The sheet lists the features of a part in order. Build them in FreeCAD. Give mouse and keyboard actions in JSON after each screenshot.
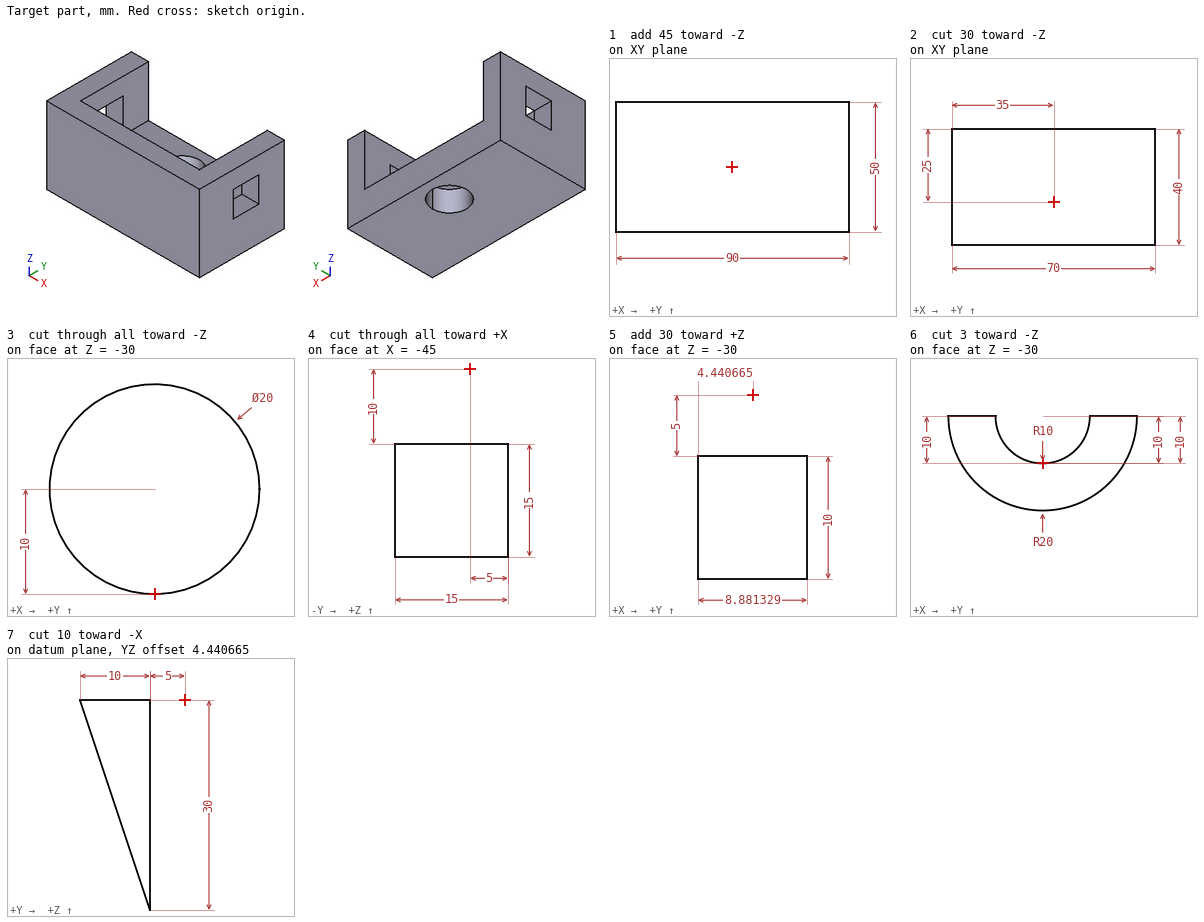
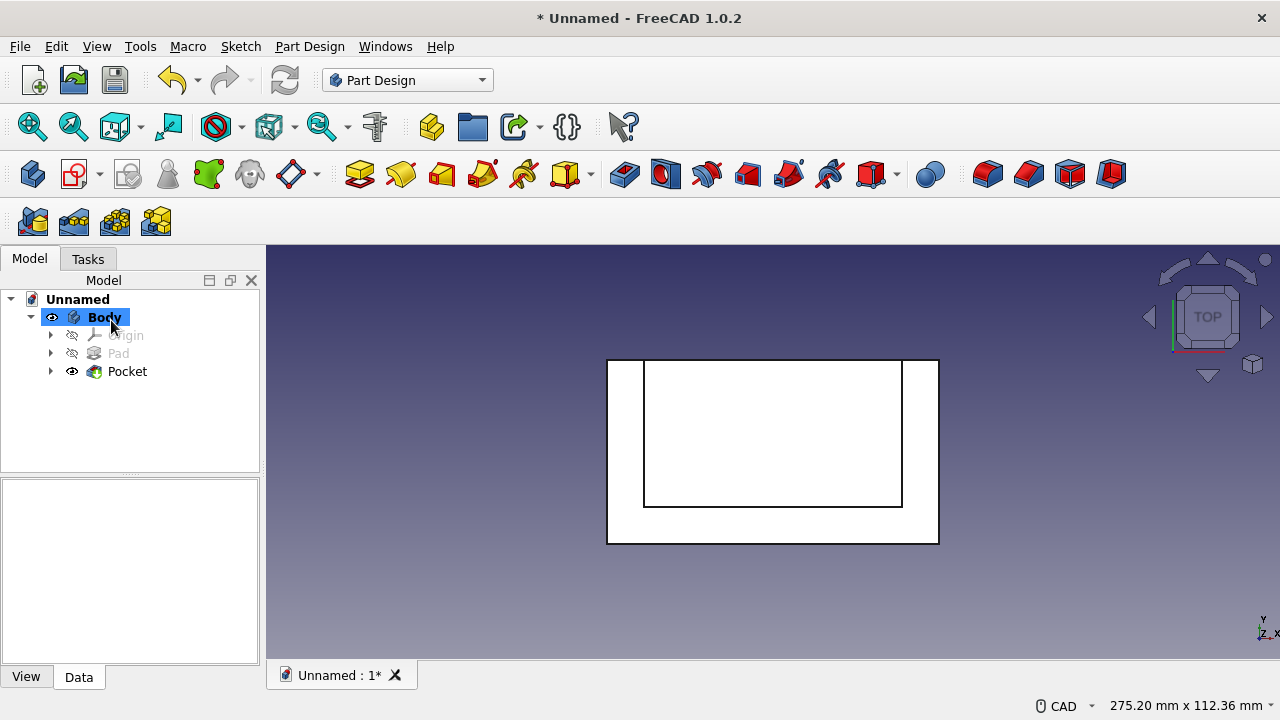
{"action": "key", "text": "v f"}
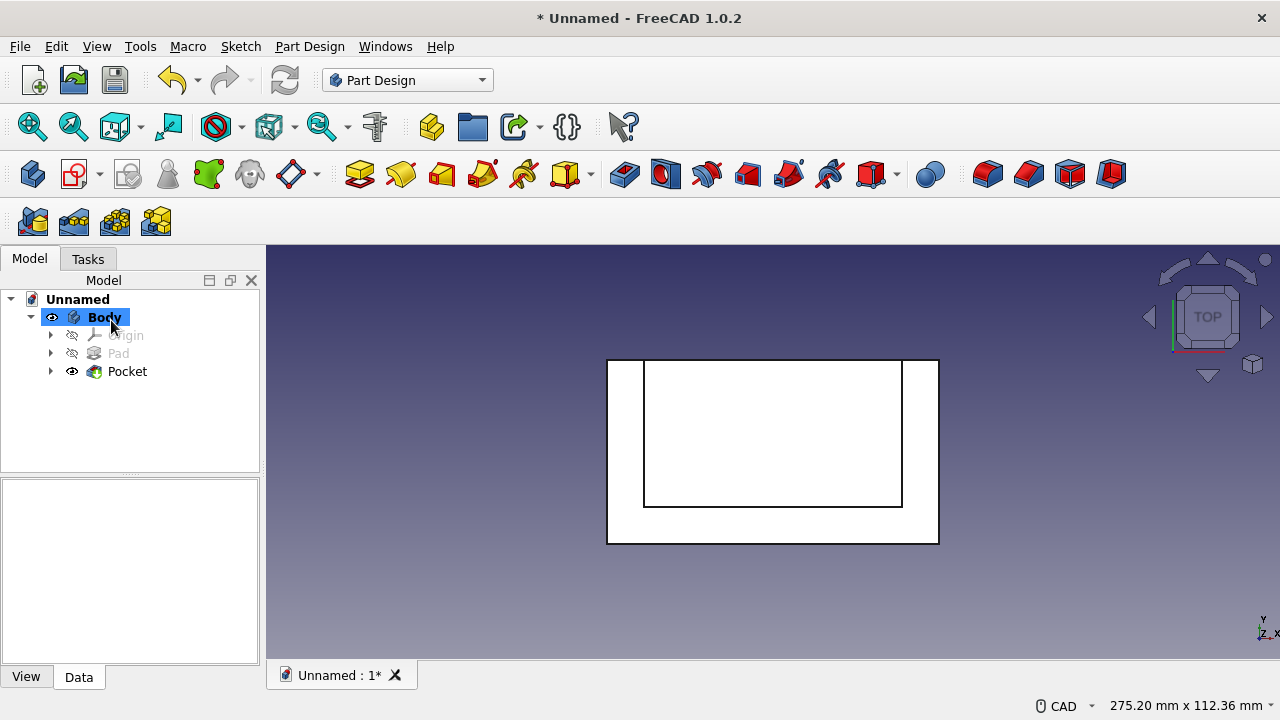
{"action": "left_click", "coordinate": [810, 433]}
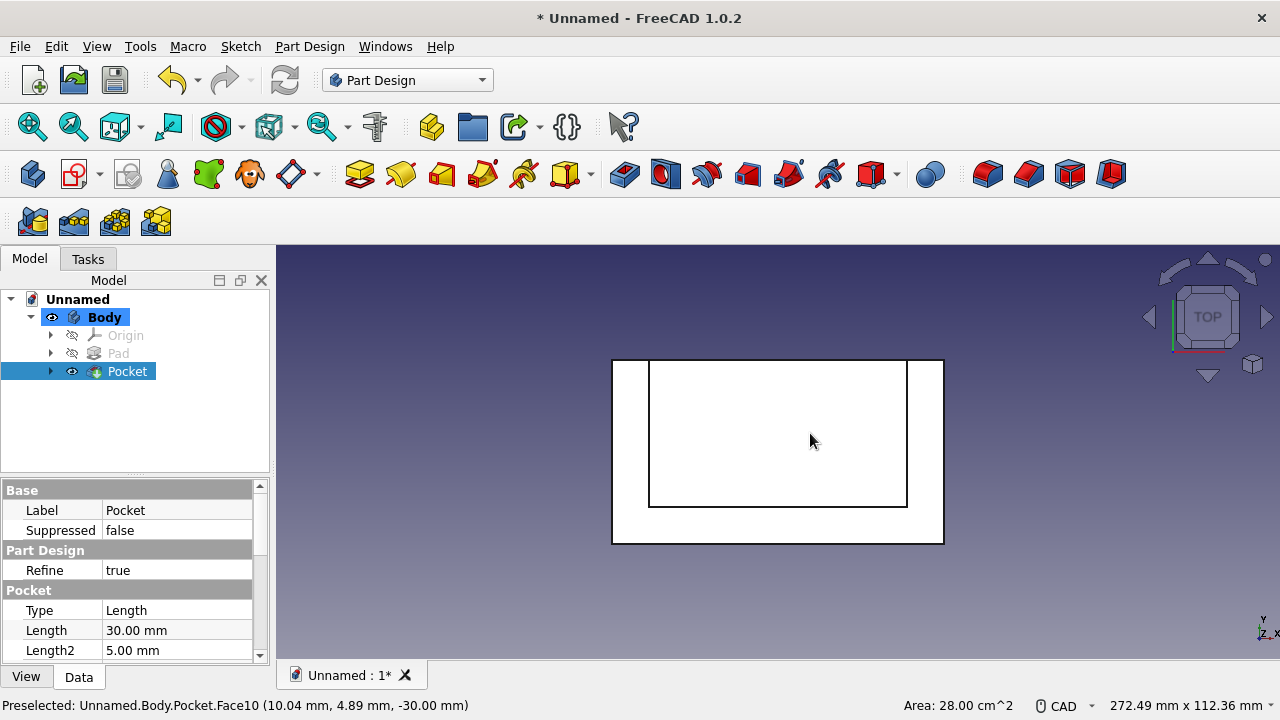
{"action": "left_click", "coordinate": [74, 174]}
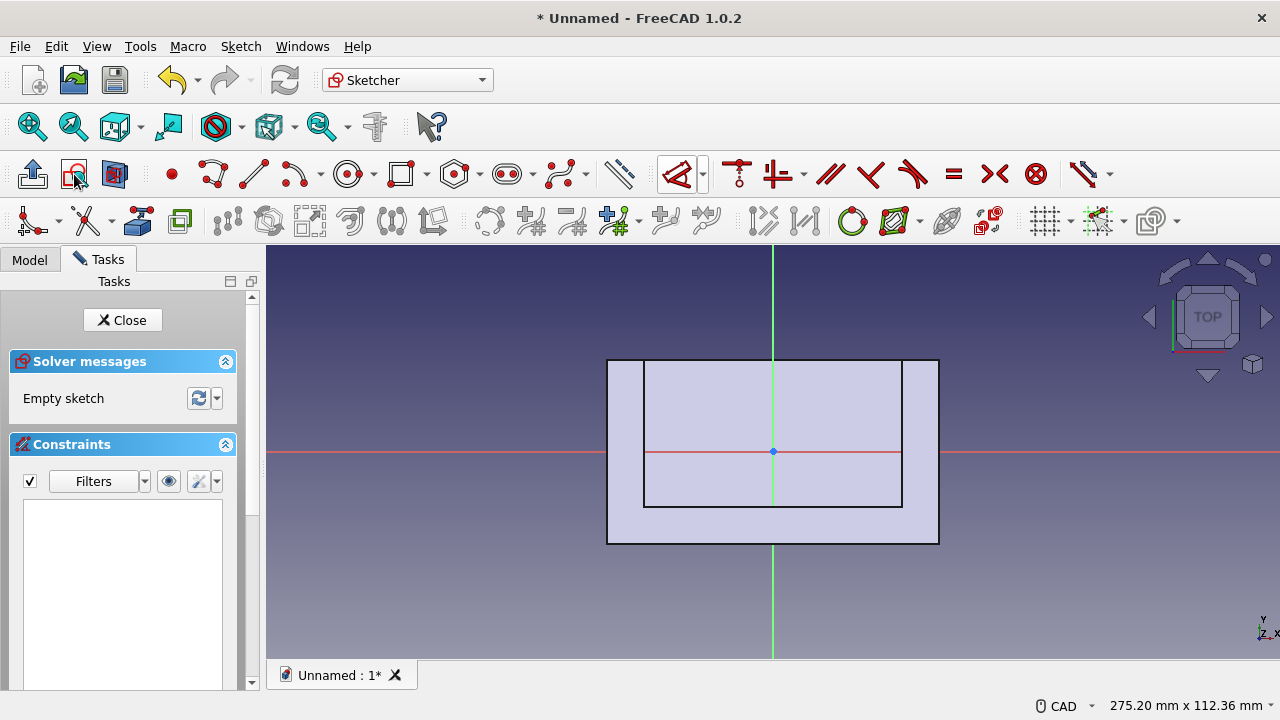
{"action": "scroll", "coordinate": [803, 399], "scroll_direction": "up", "scroll_amount": 6}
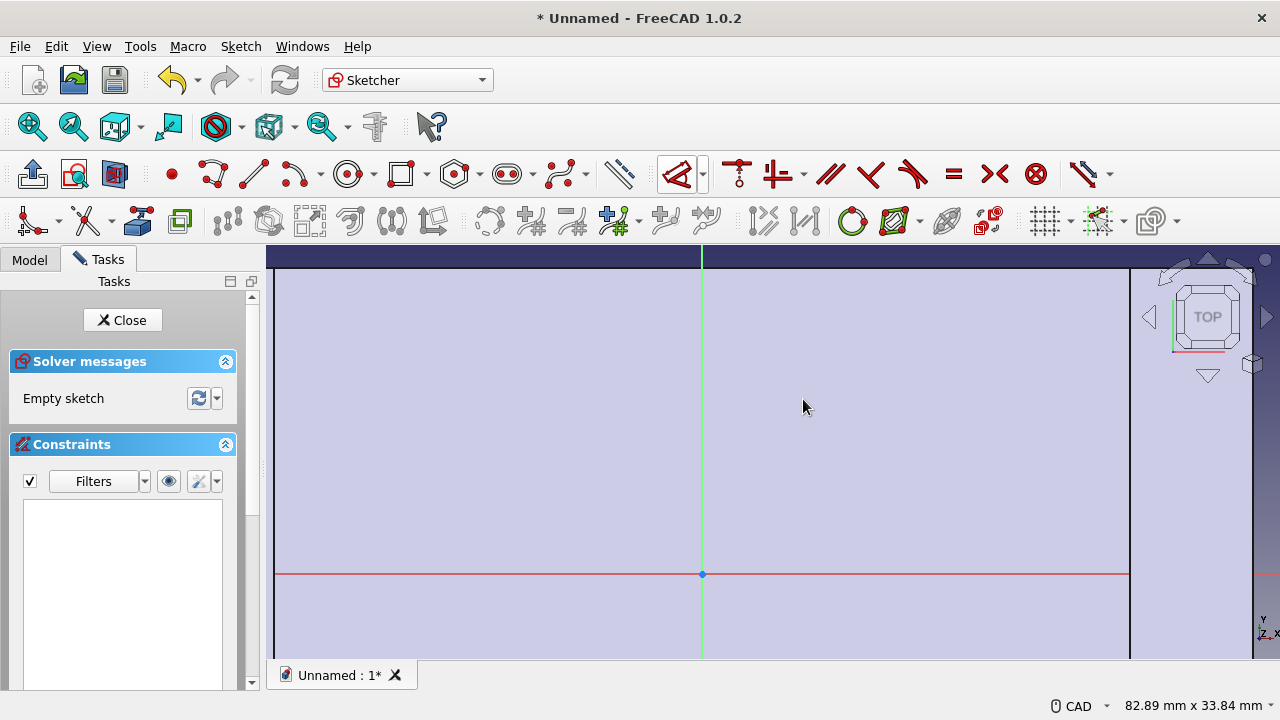
{"action": "key", "text": "g c"}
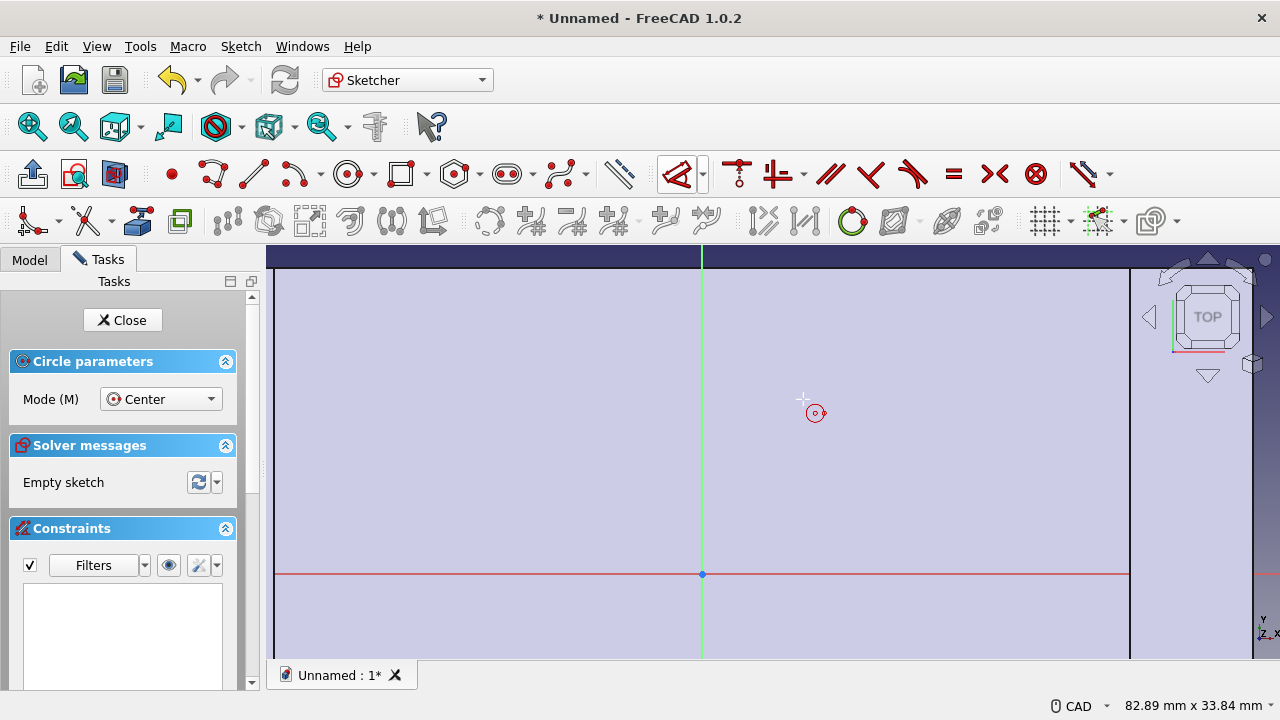
{"action": "left_click", "coordinate": [702, 452]}
{"action": "mouse_move", "coordinate": [789, 365]}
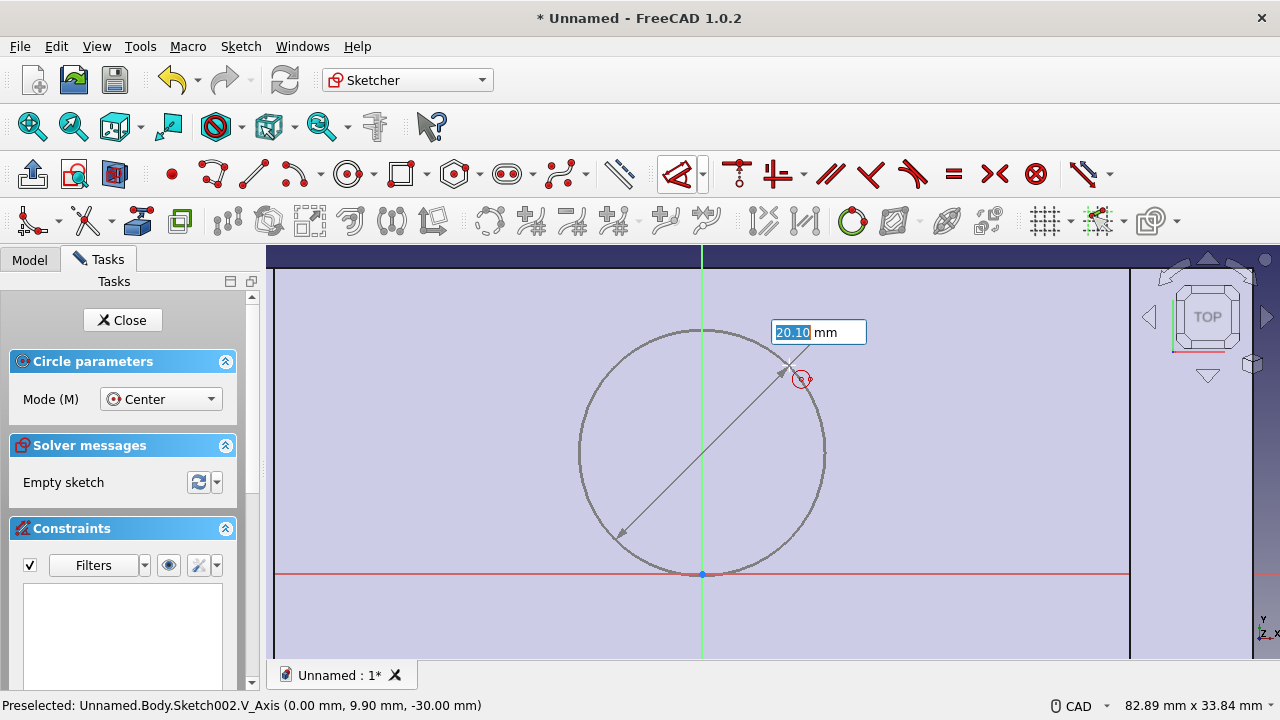
{"action": "type", "text": "20"}
{"action": "key", "text": "Return"}
{"action": "key", "text": "Escape"}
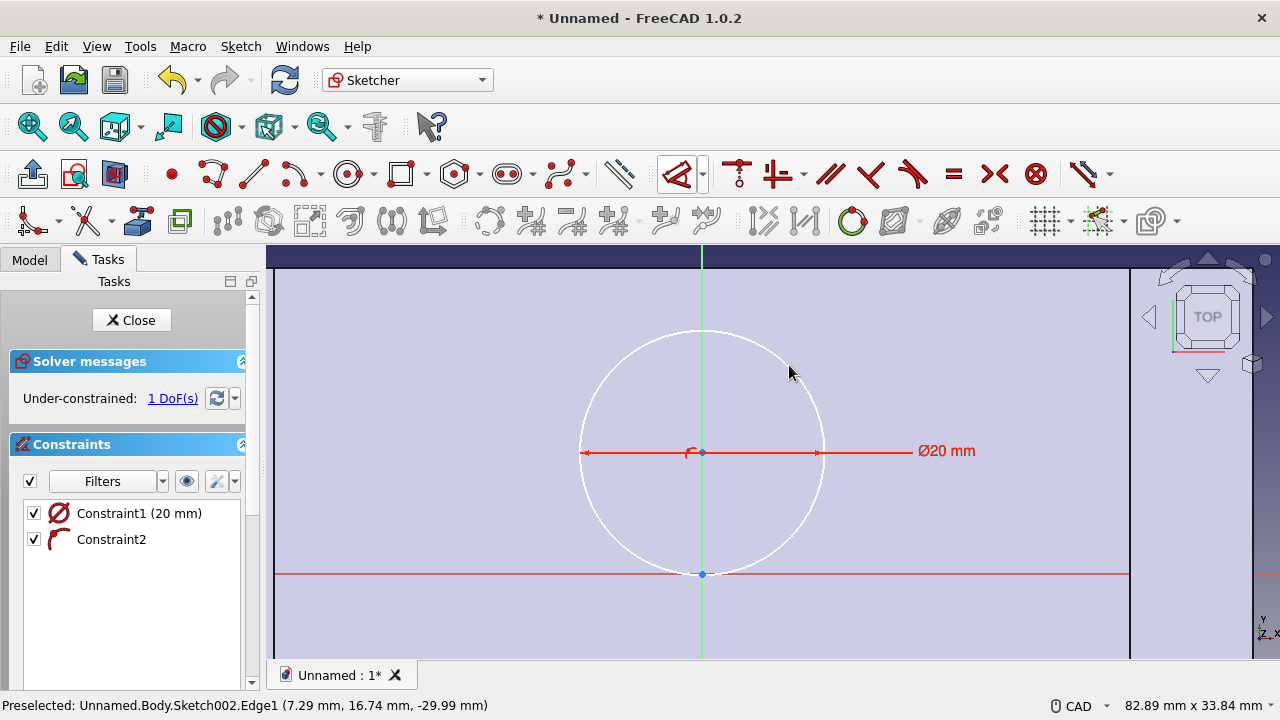
{"action": "left_click", "coordinate": [702, 453]}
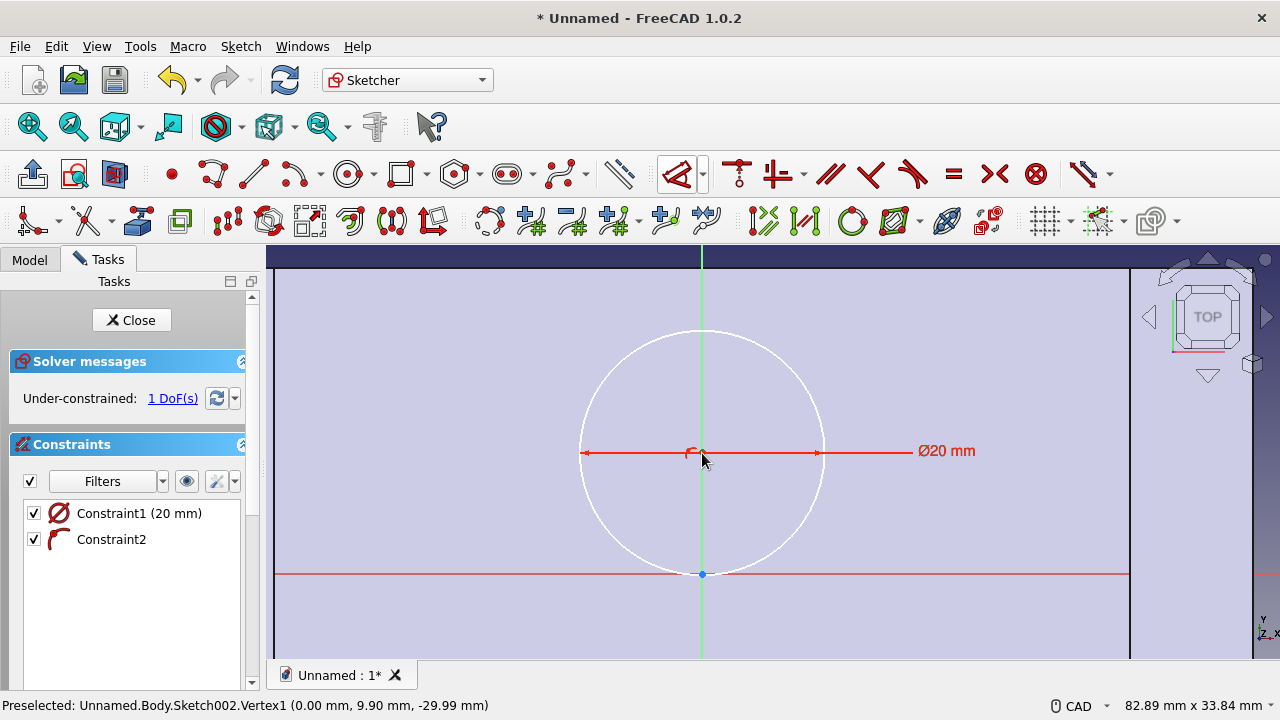
{"action": "key", "text": "i"}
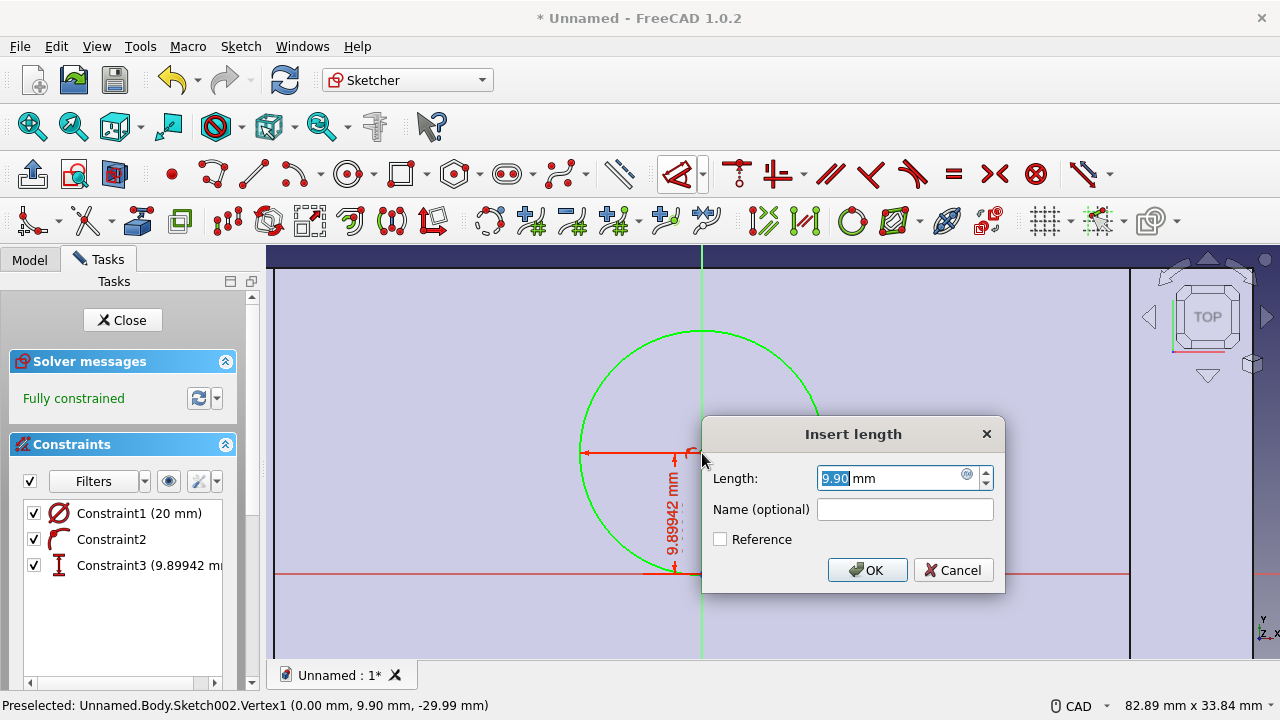
{"action": "type", "text": "10"}
{"action": "key", "text": "Return"}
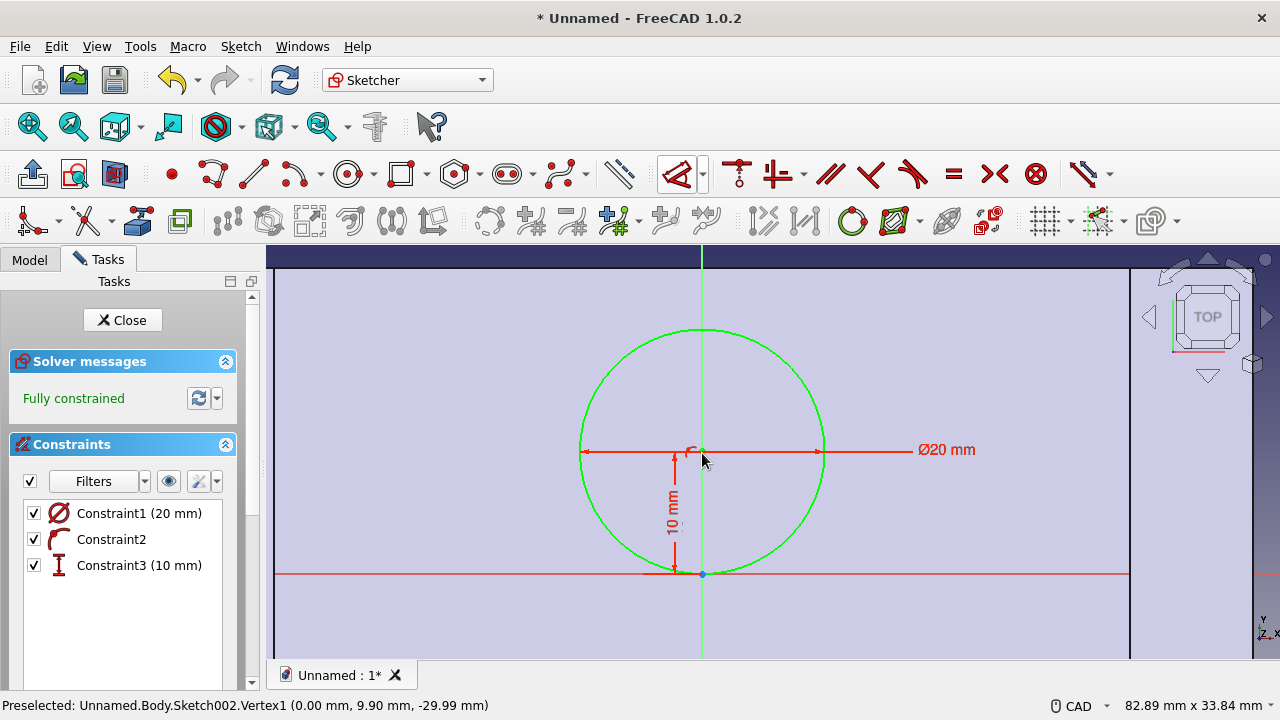
{"action": "left_click", "coordinate": [123, 320]}